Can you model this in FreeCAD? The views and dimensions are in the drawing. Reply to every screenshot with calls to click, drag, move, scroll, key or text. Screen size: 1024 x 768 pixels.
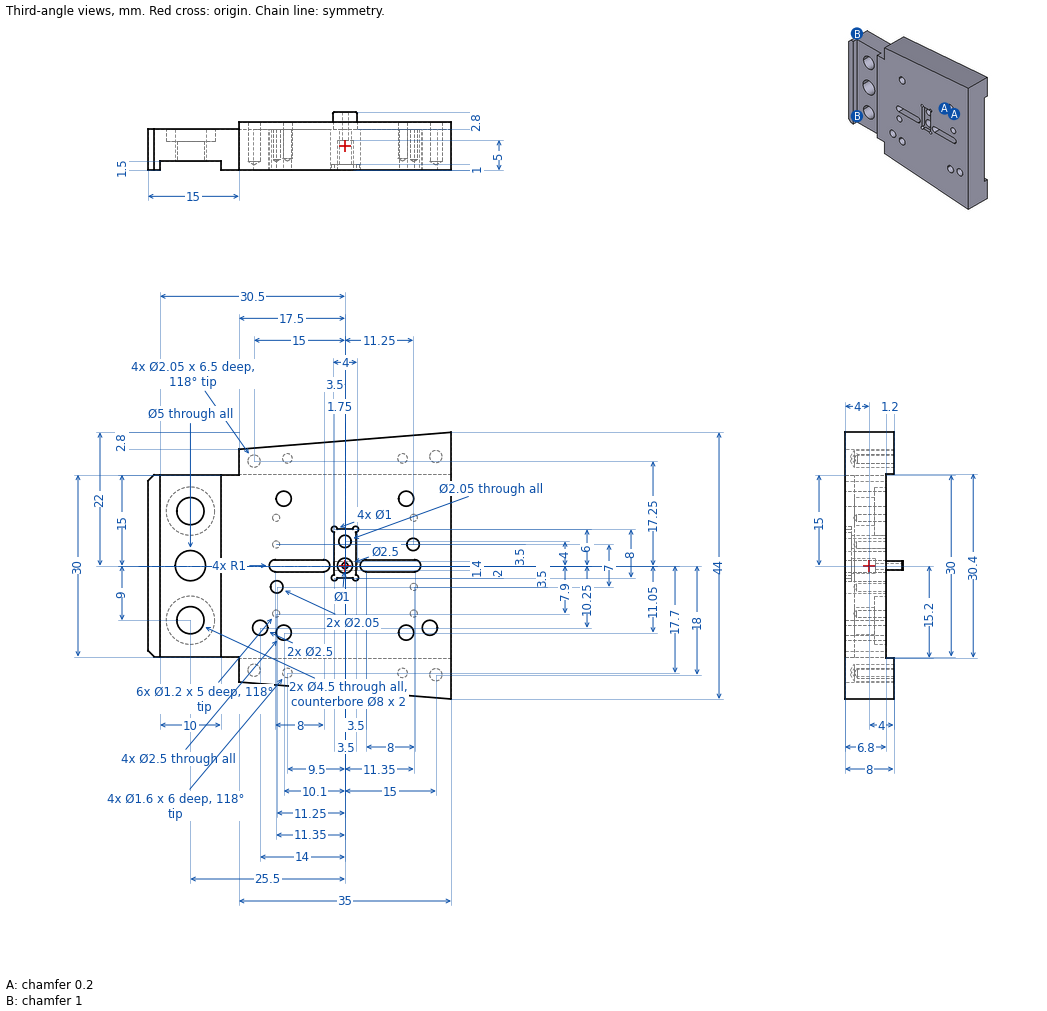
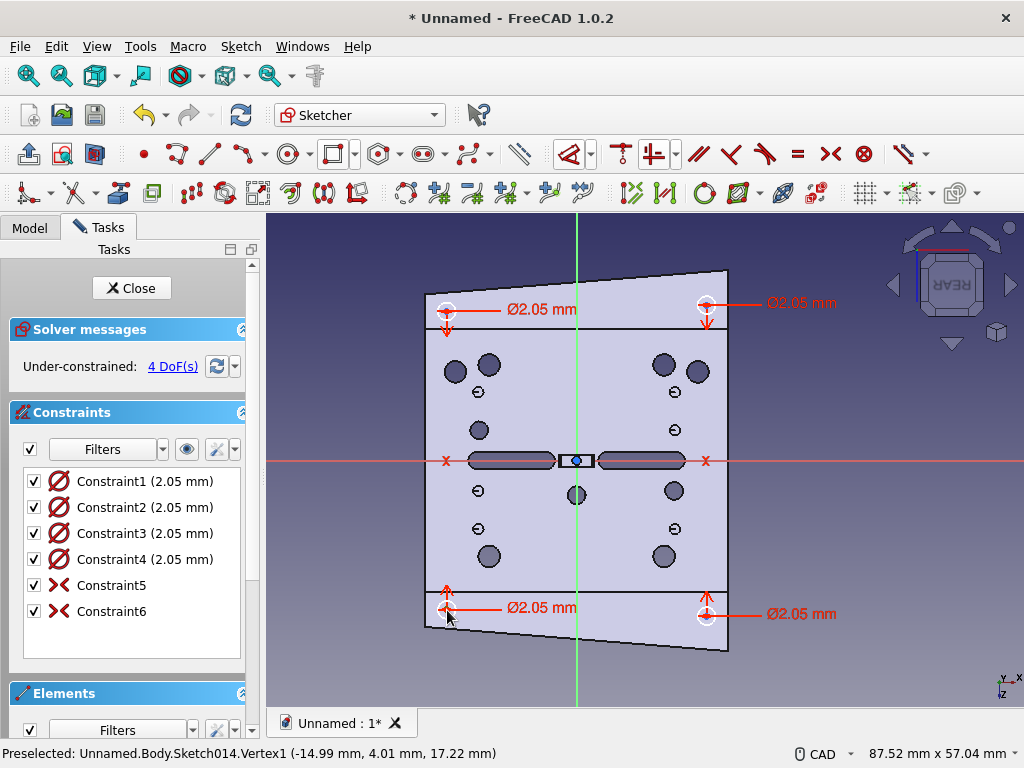
key(l)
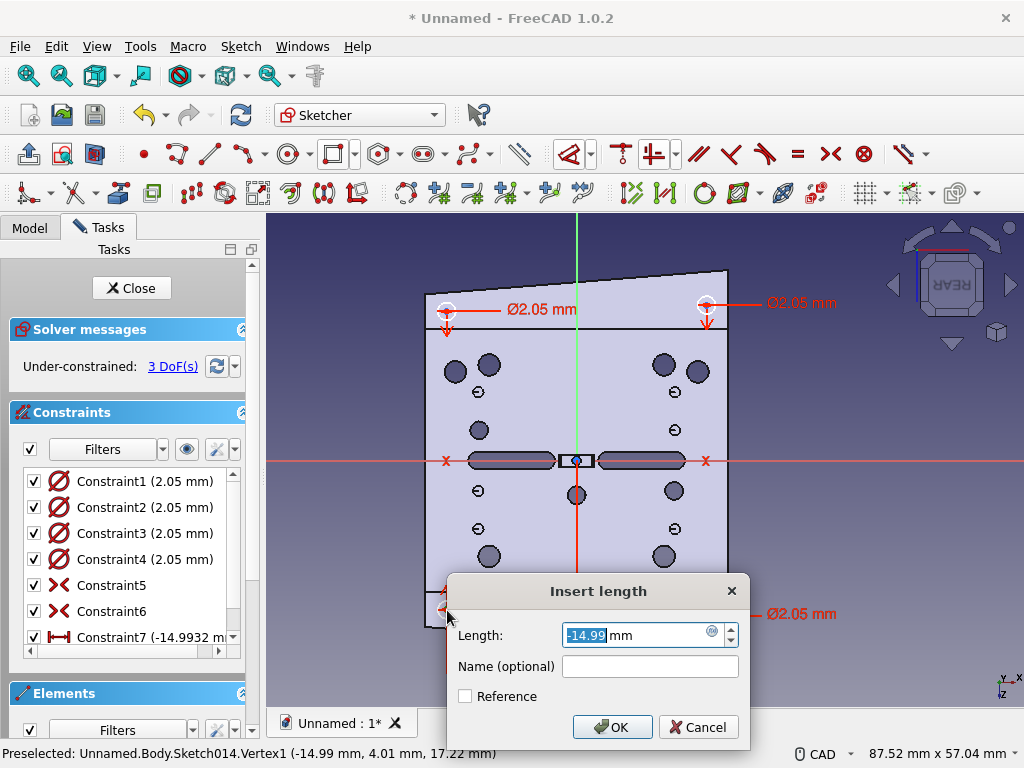
text(-15)
key(Return)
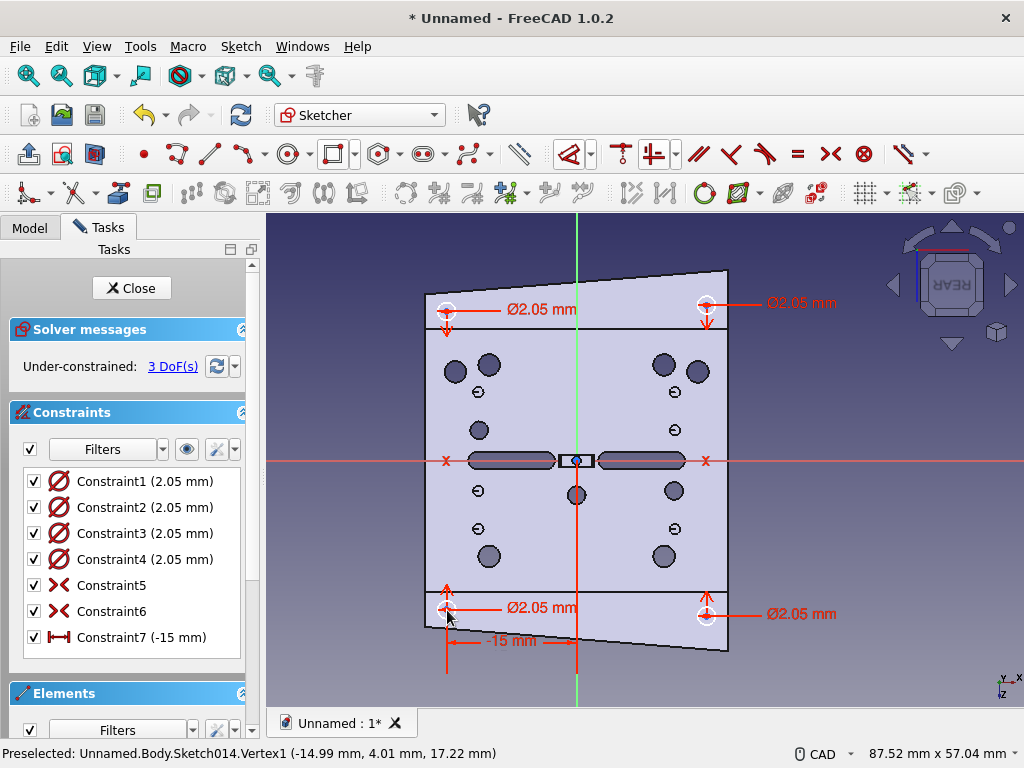
click(707, 305)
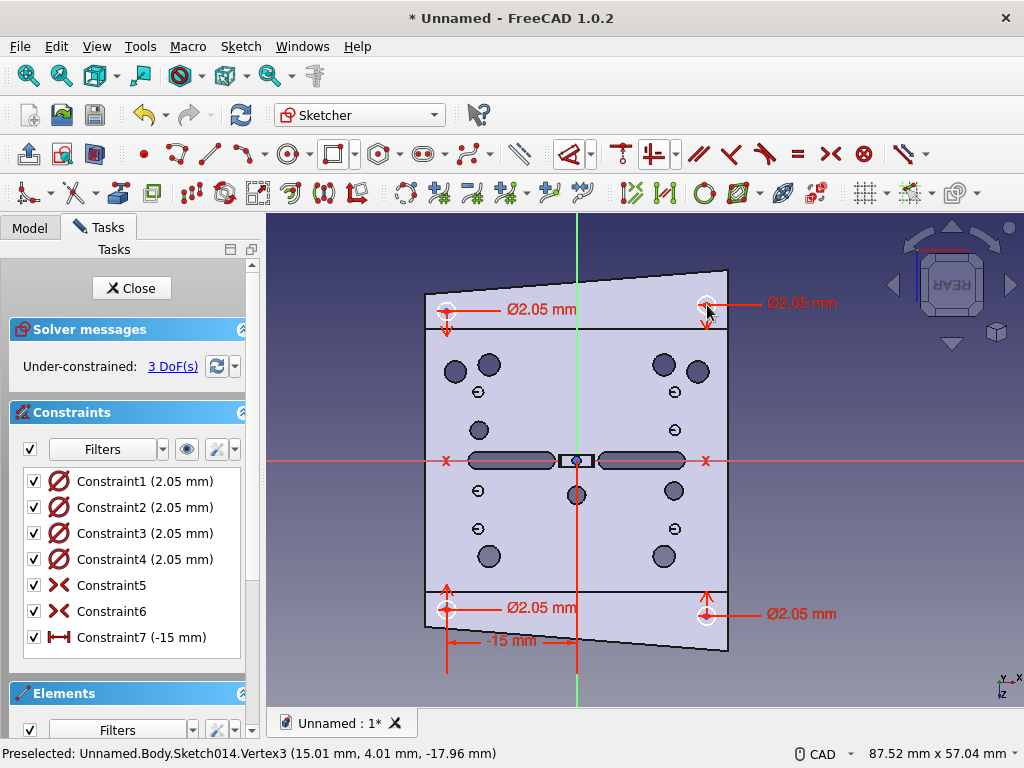
click(590, 154)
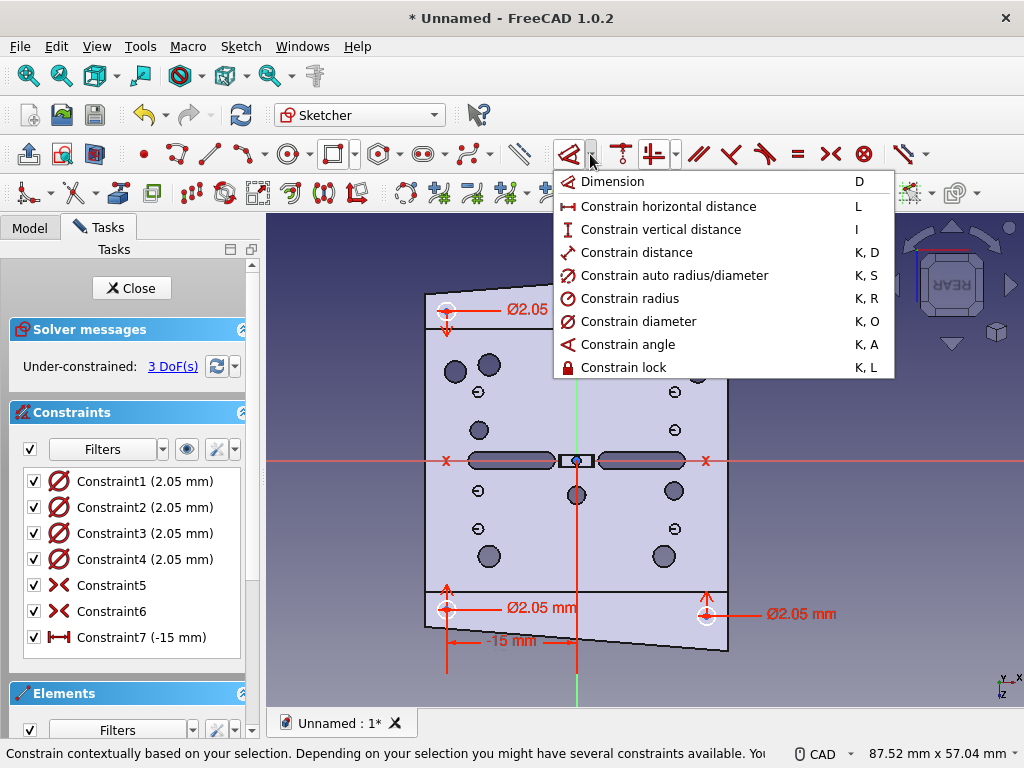
click(724, 206)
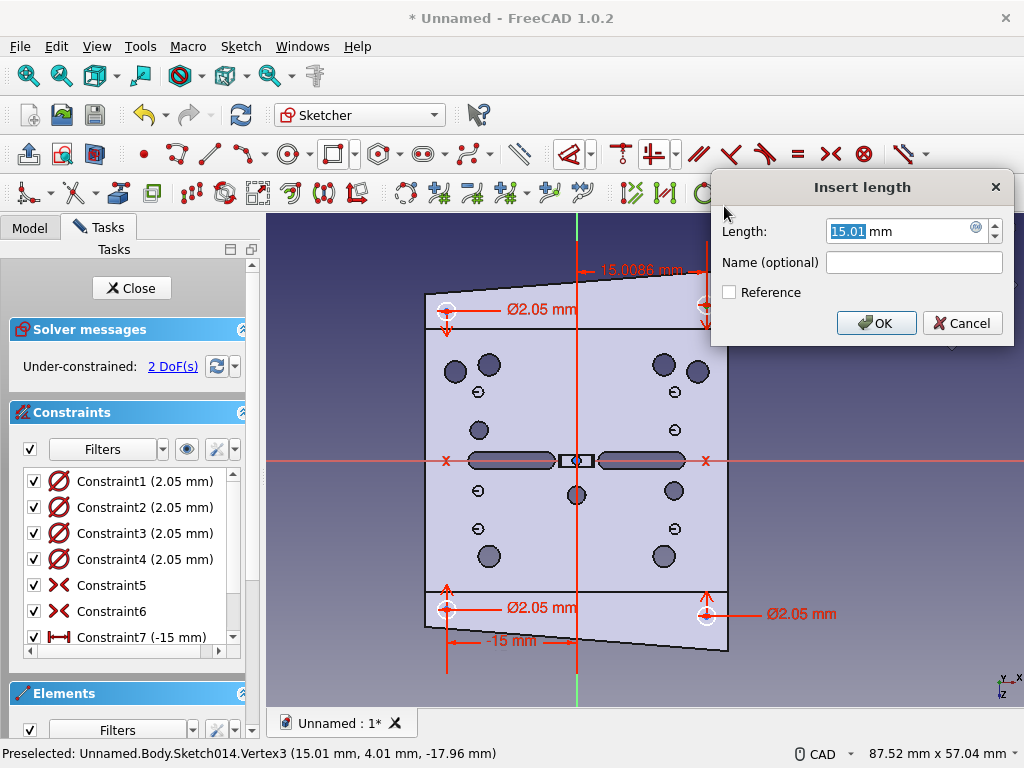
text(15)
key(Return)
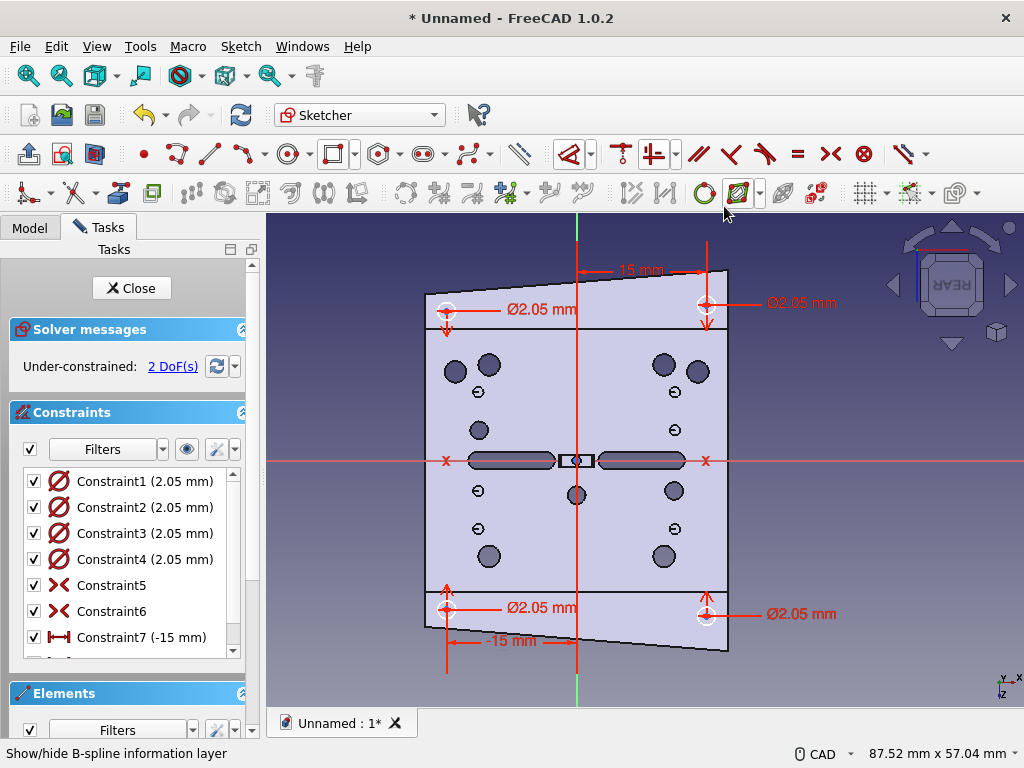
click(707, 305)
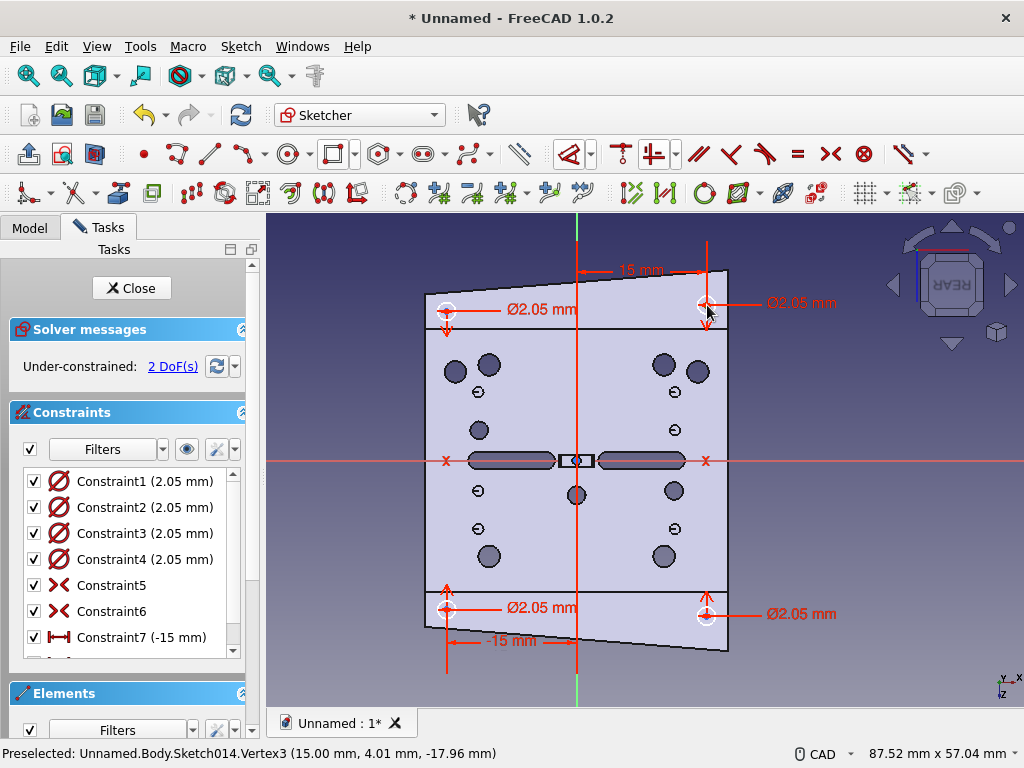
key(i)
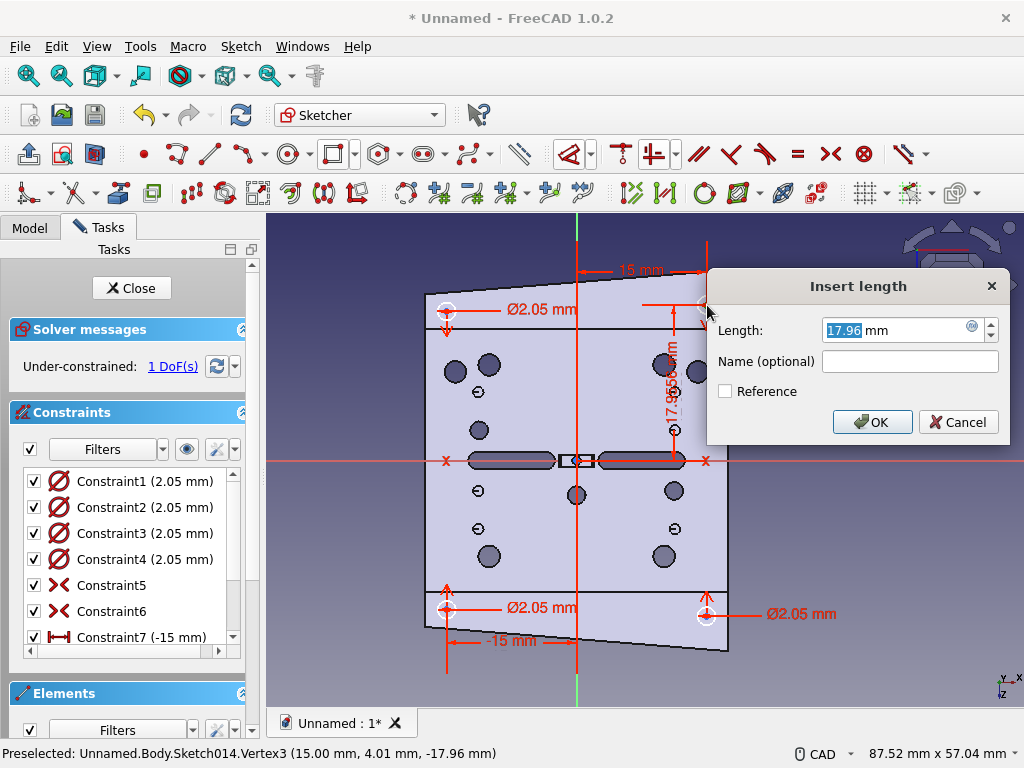
text(18)
key(Return)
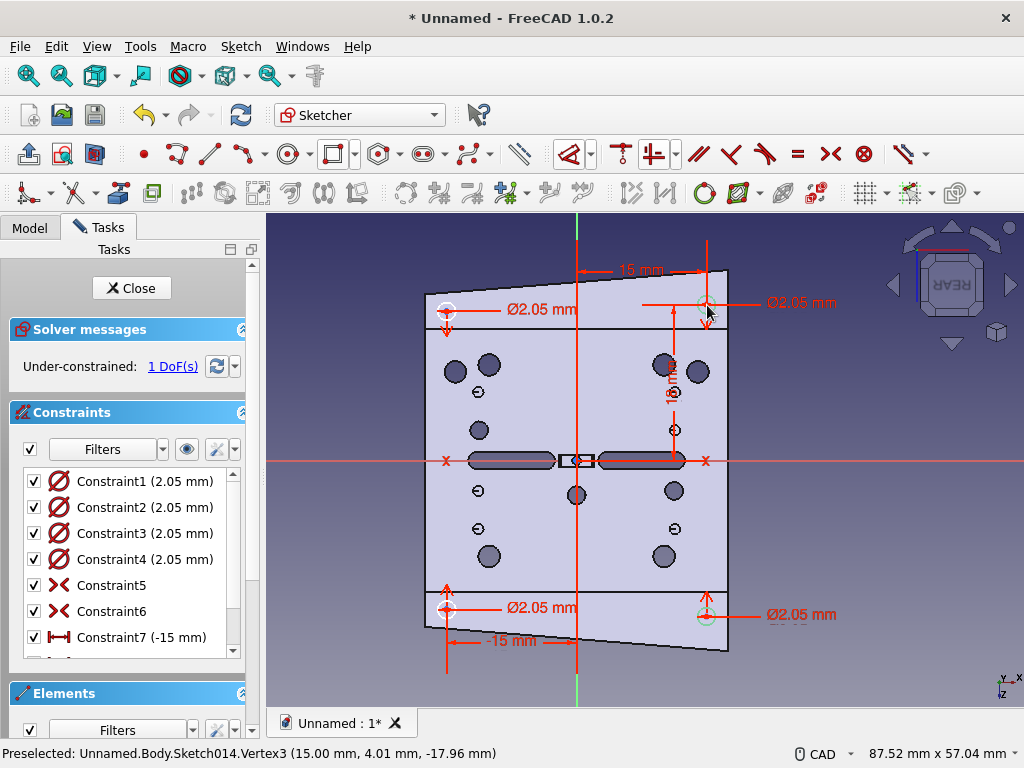
click(447, 610)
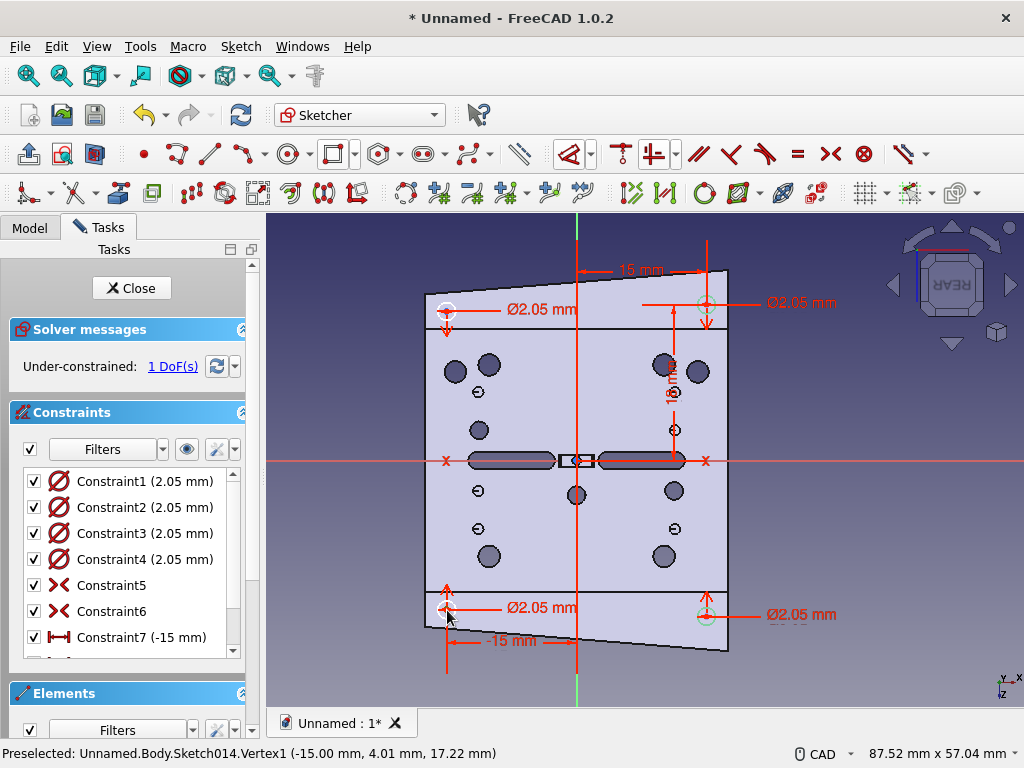
key(i)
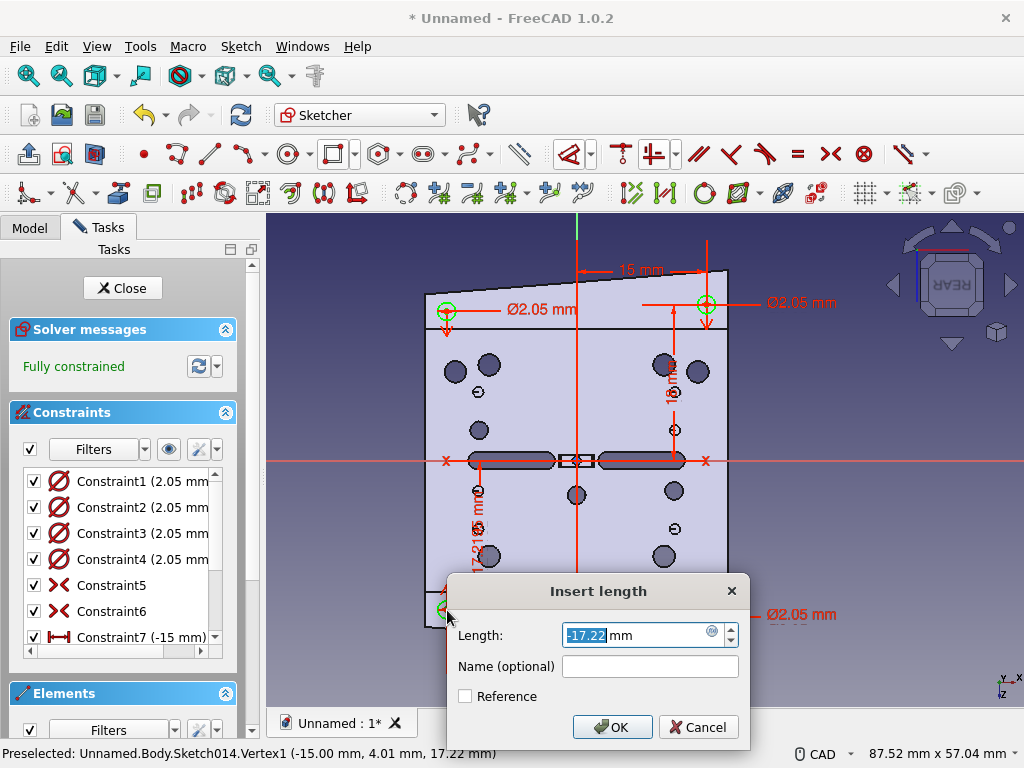
text(-17.25)
key(Return)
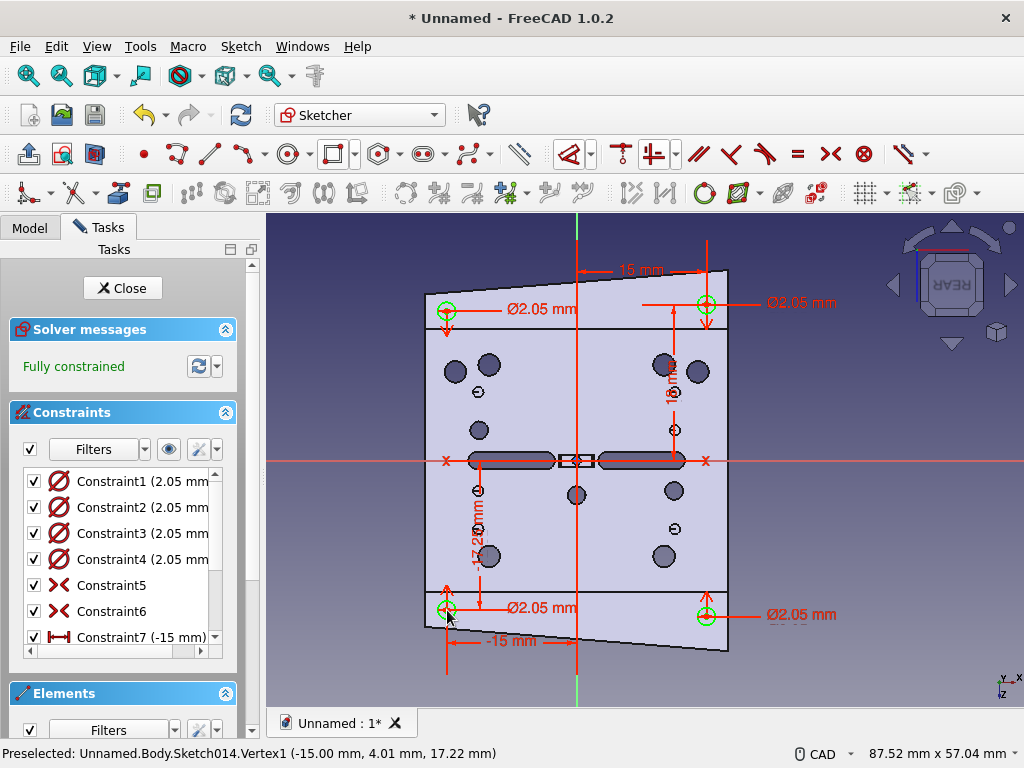
click(123, 288)